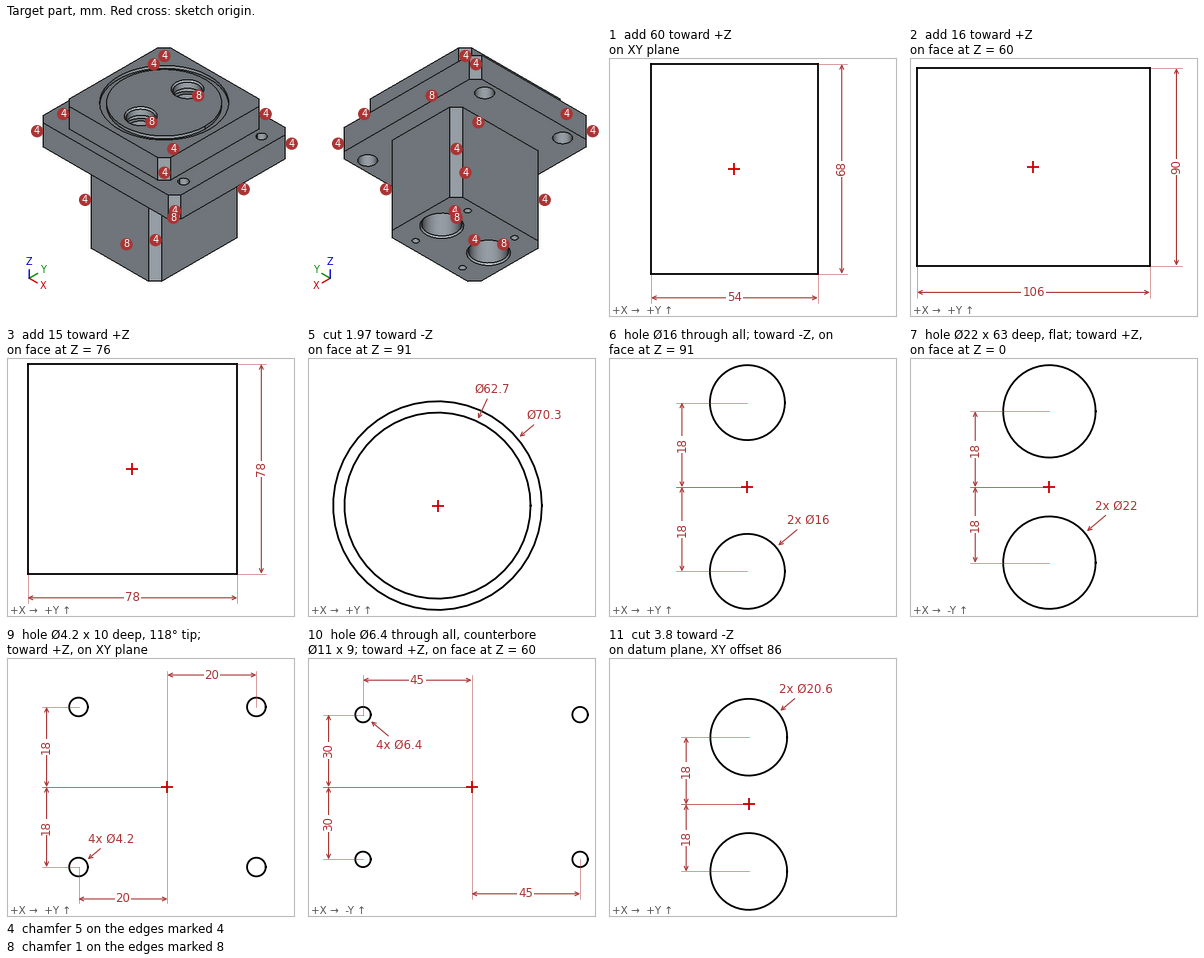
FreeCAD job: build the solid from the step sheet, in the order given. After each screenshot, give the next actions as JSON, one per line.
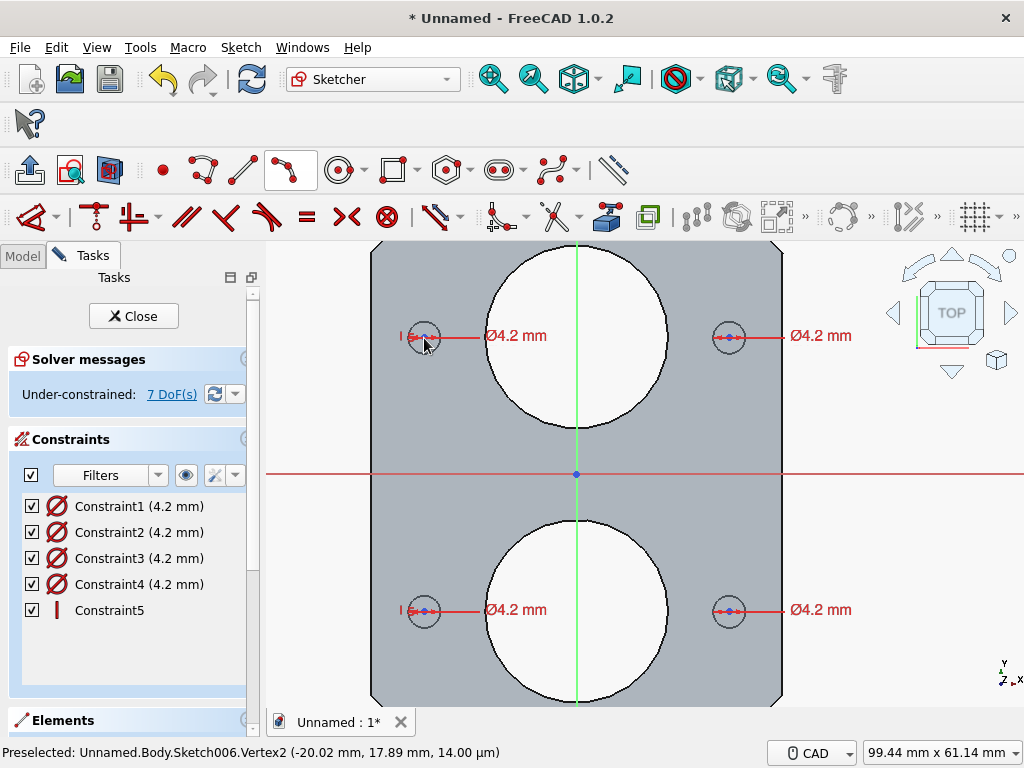
{"action": "left_click", "coordinate": [424, 338]}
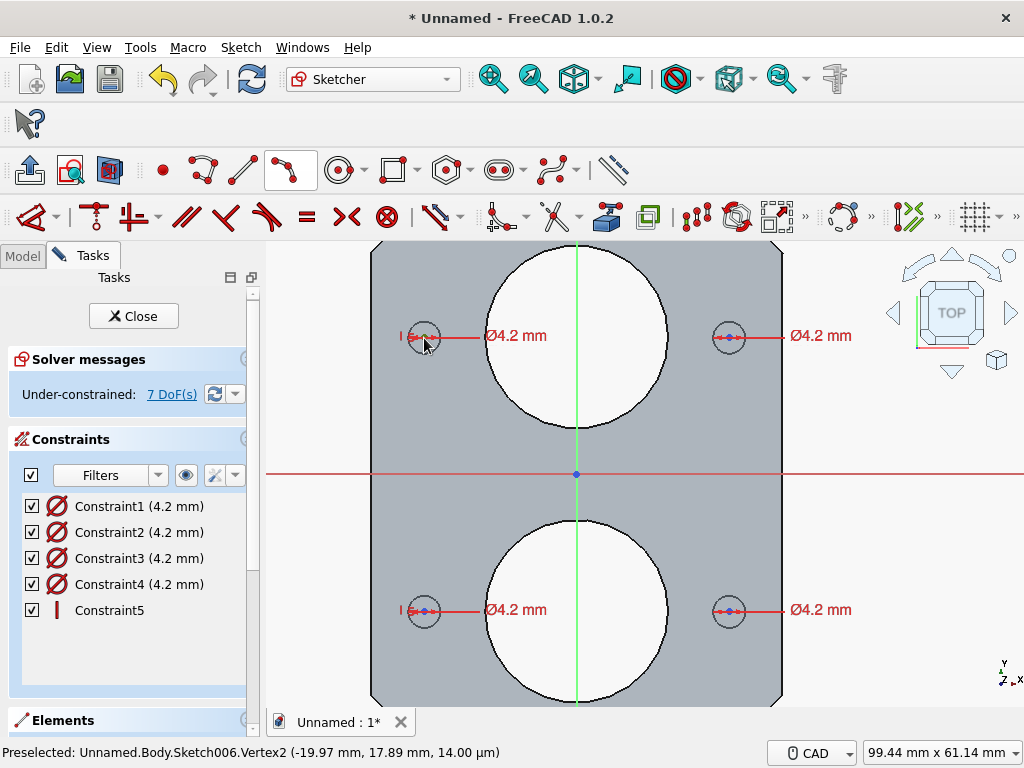
{"action": "left_click", "coordinate": [729, 338]}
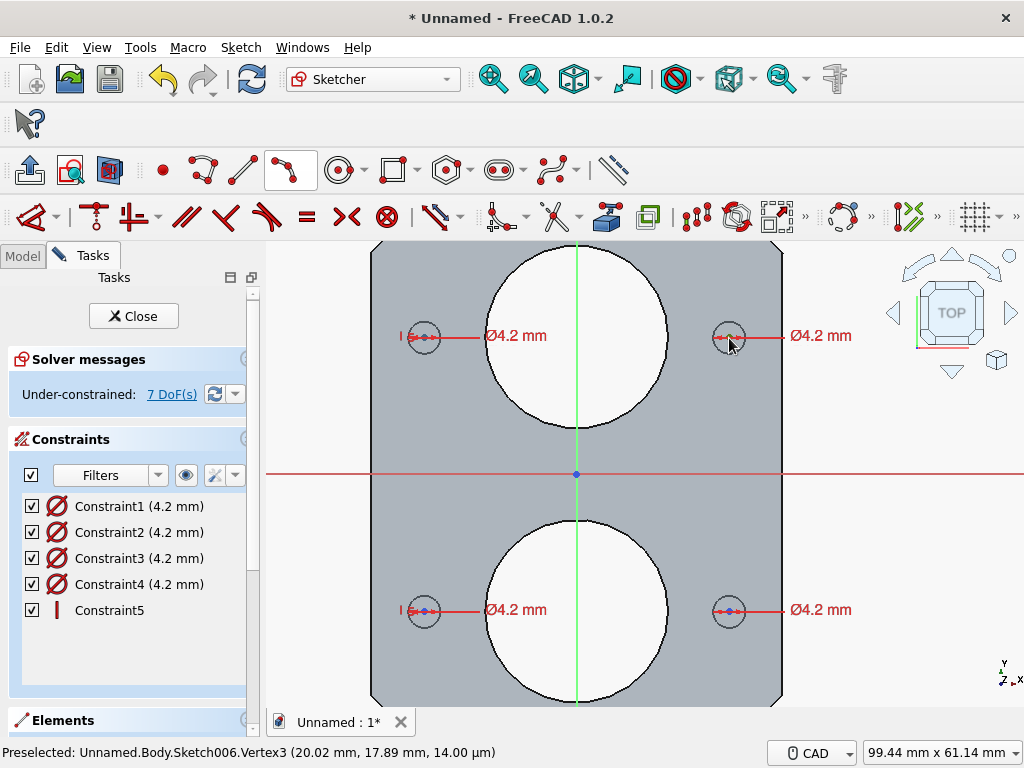
{"action": "key", "text": "h"}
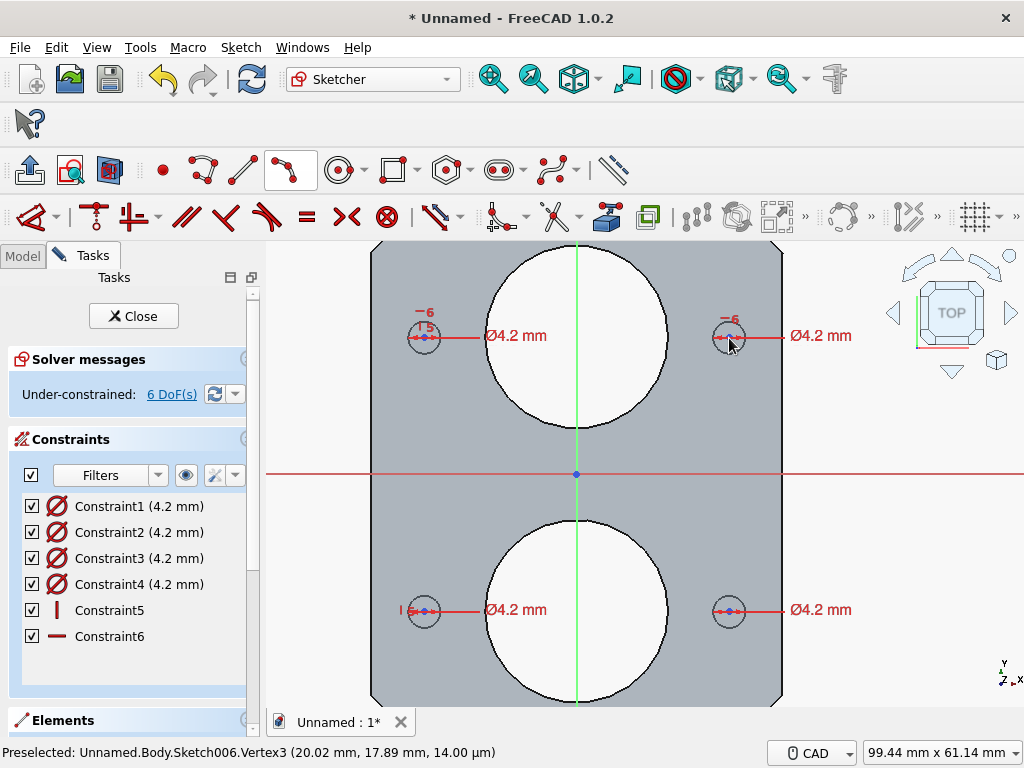
{"action": "left_click", "coordinate": [729, 338]}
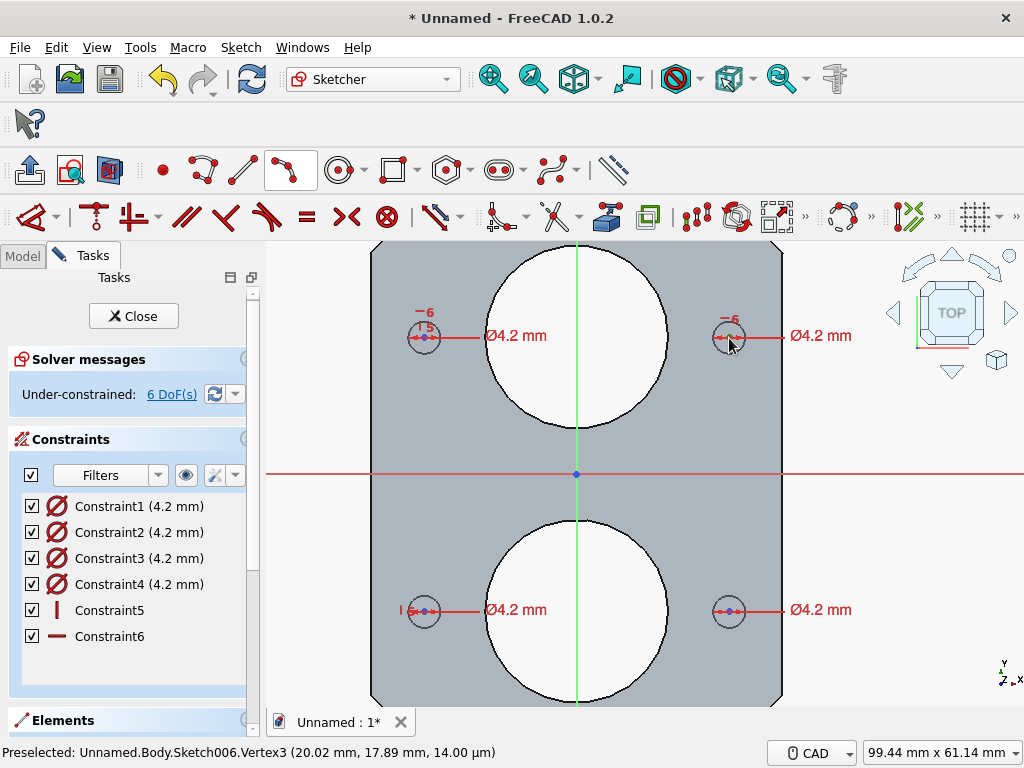
{"action": "left_click", "coordinate": [729, 612]}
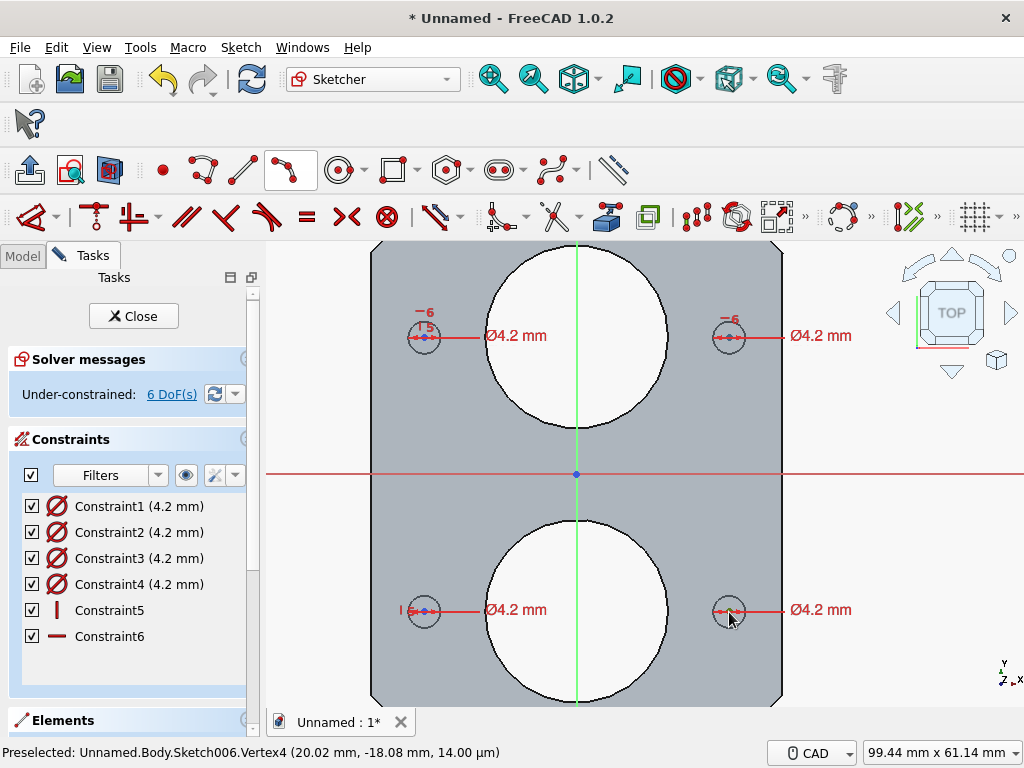
{"action": "key", "text": "v"}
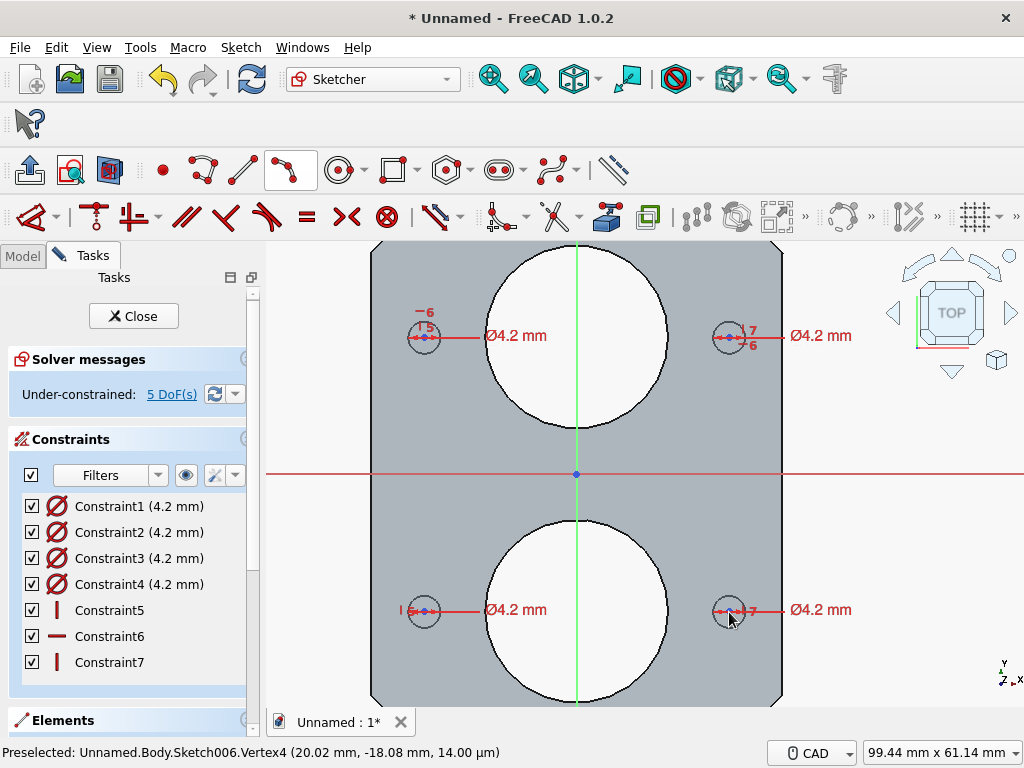
{"action": "left_click", "coordinate": [424, 612]}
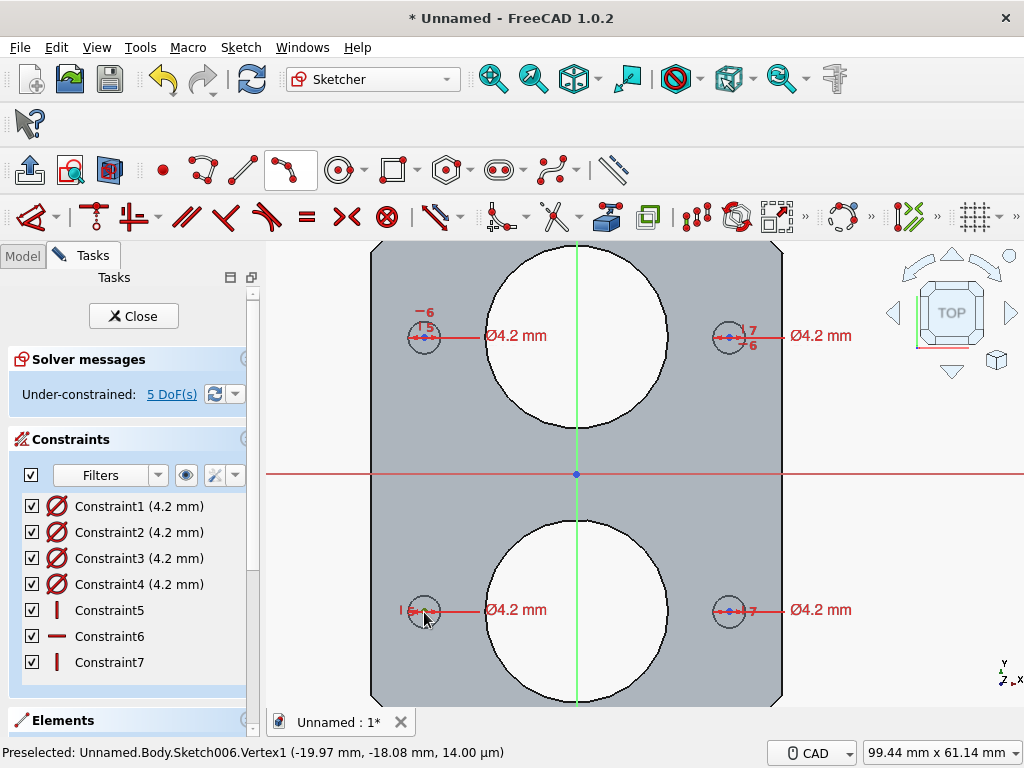
{"action": "left_click", "coordinate": [729, 612]}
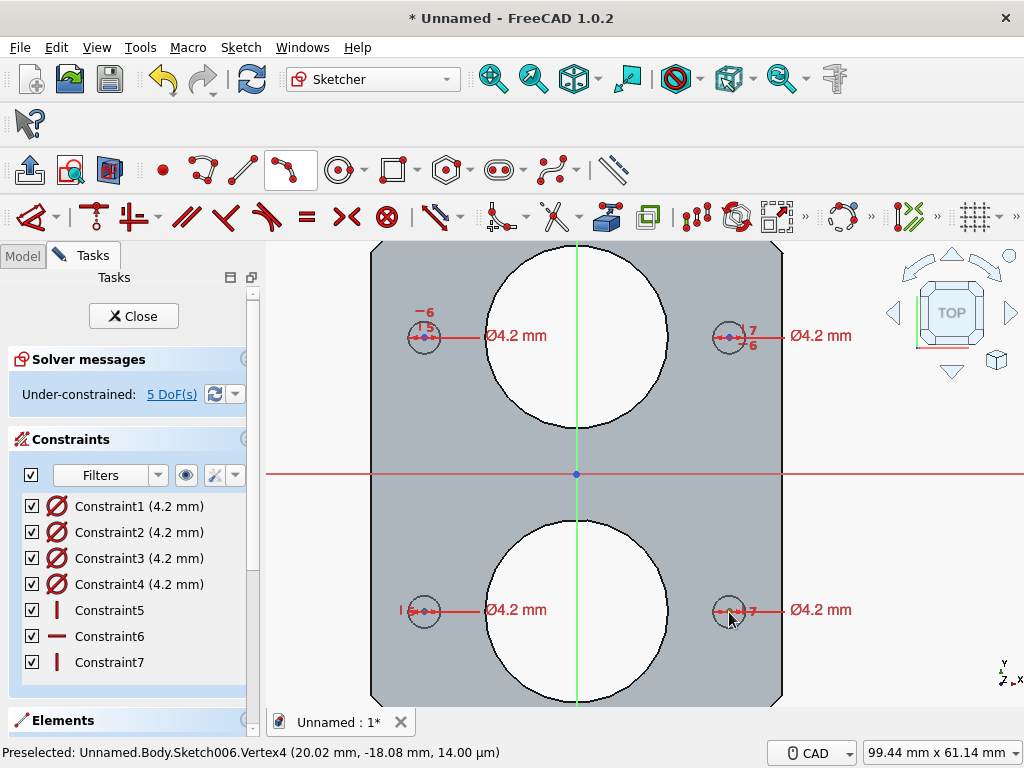
{"action": "key", "text": "h"}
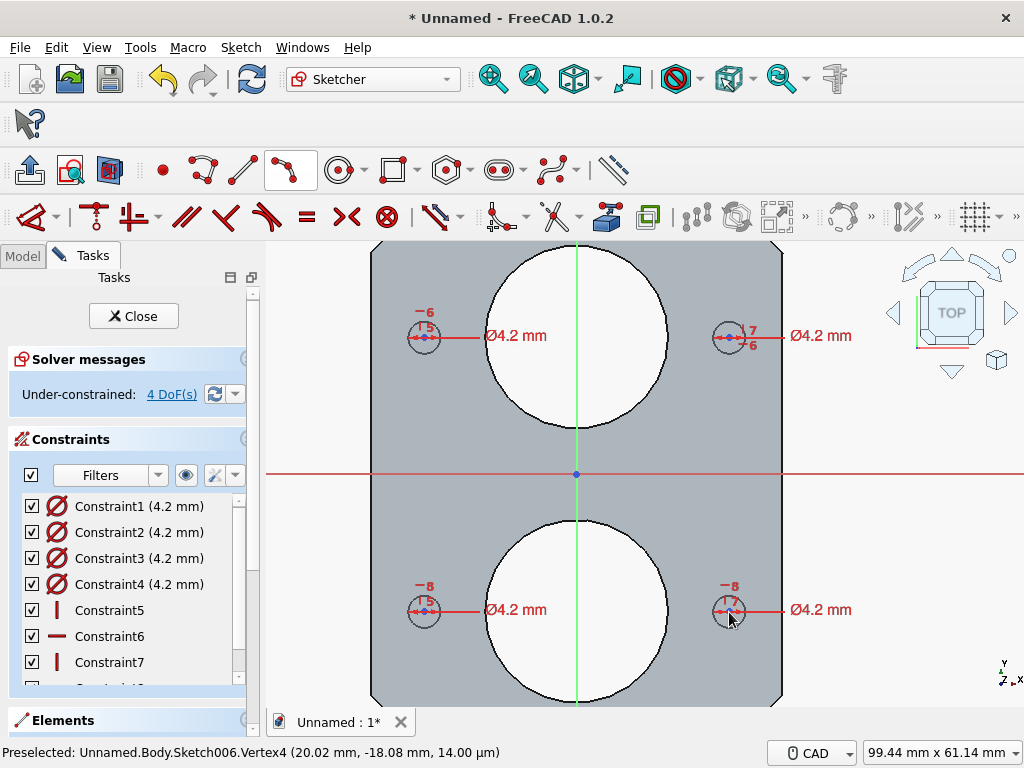
{"action": "left_click", "coordinate": [32, 218]}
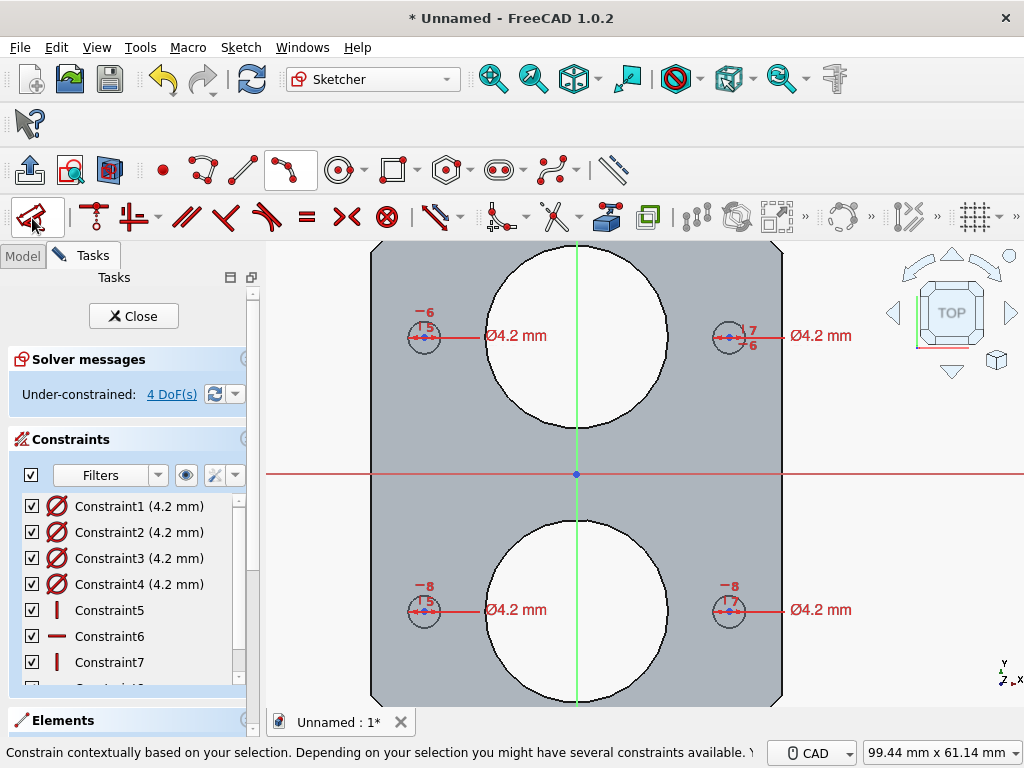
{"action": "left_click", "coordinate": [424, 612]}
{"action": "left_click", "coordinate": [501, 646]}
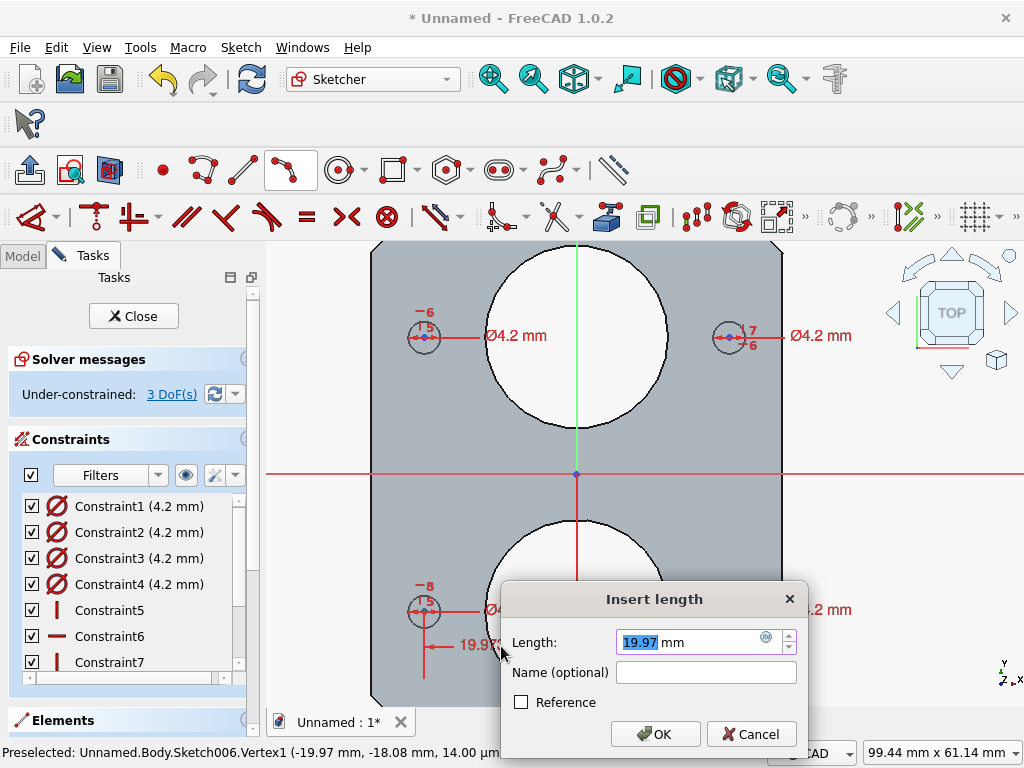
{"action": "type", "text": "20"}
{"action": "key", "text": "Return"}